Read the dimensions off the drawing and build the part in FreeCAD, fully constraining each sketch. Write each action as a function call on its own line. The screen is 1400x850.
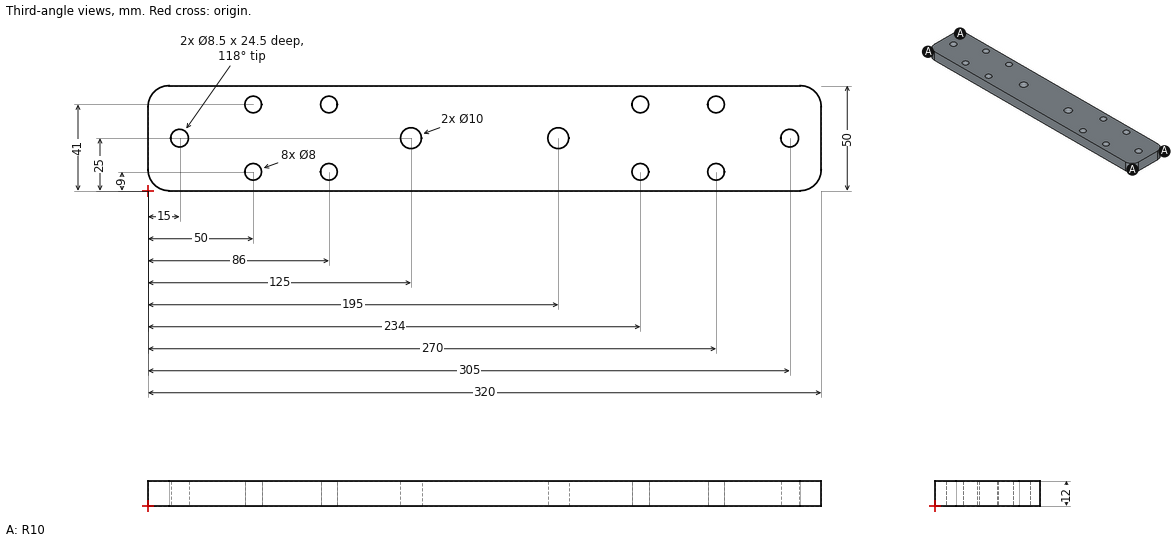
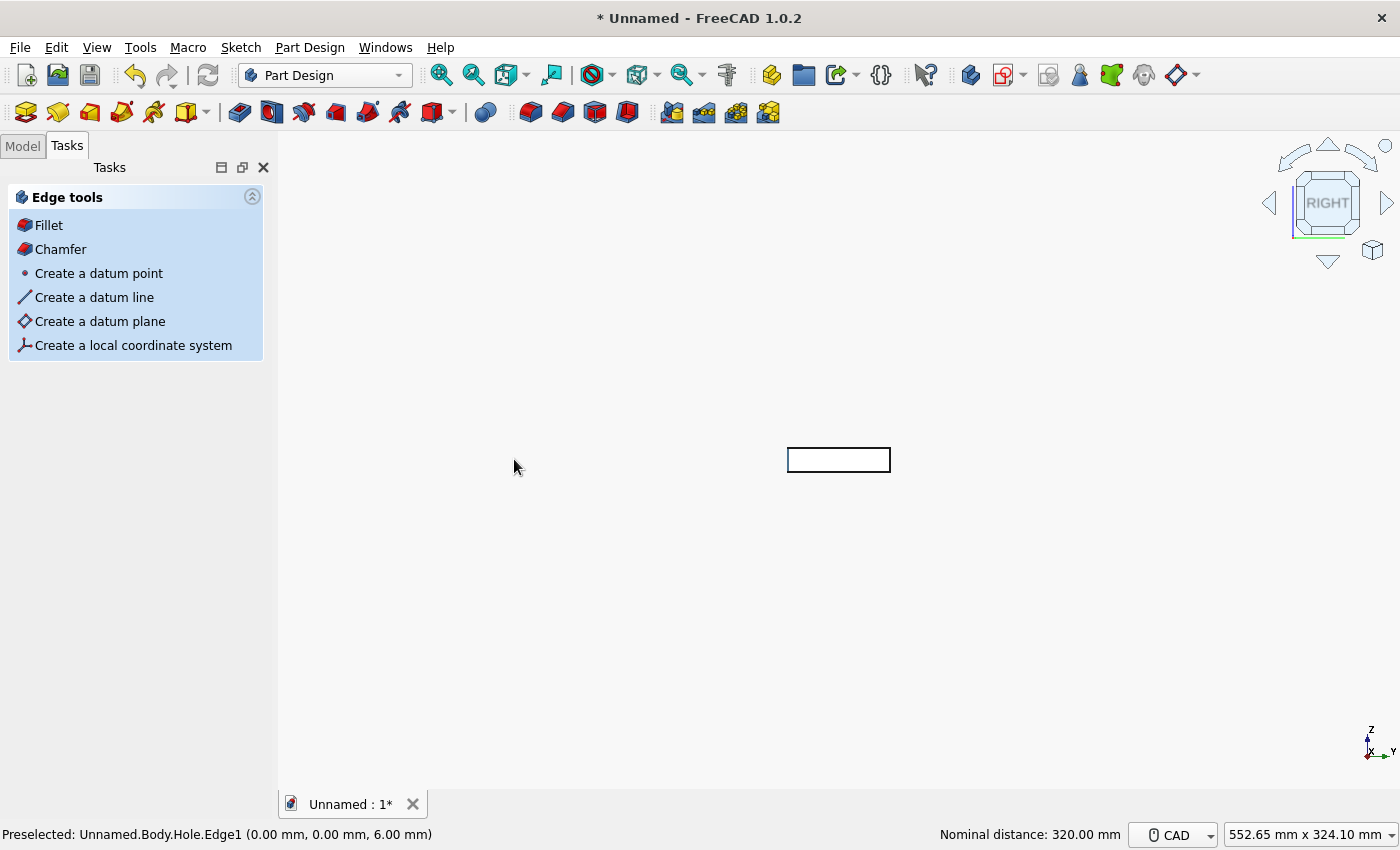
click(442, 76)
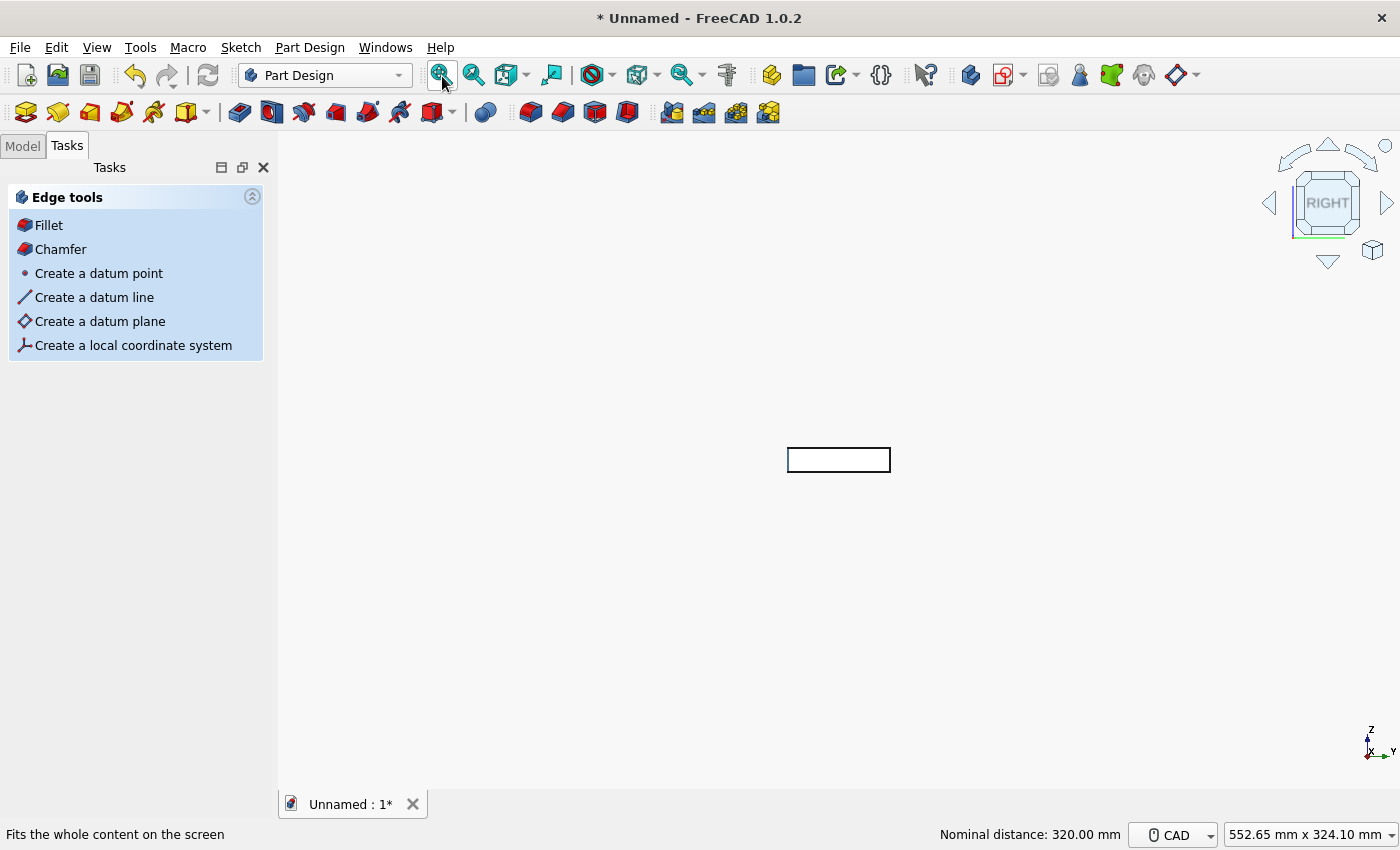
click(890, 459, ctrl)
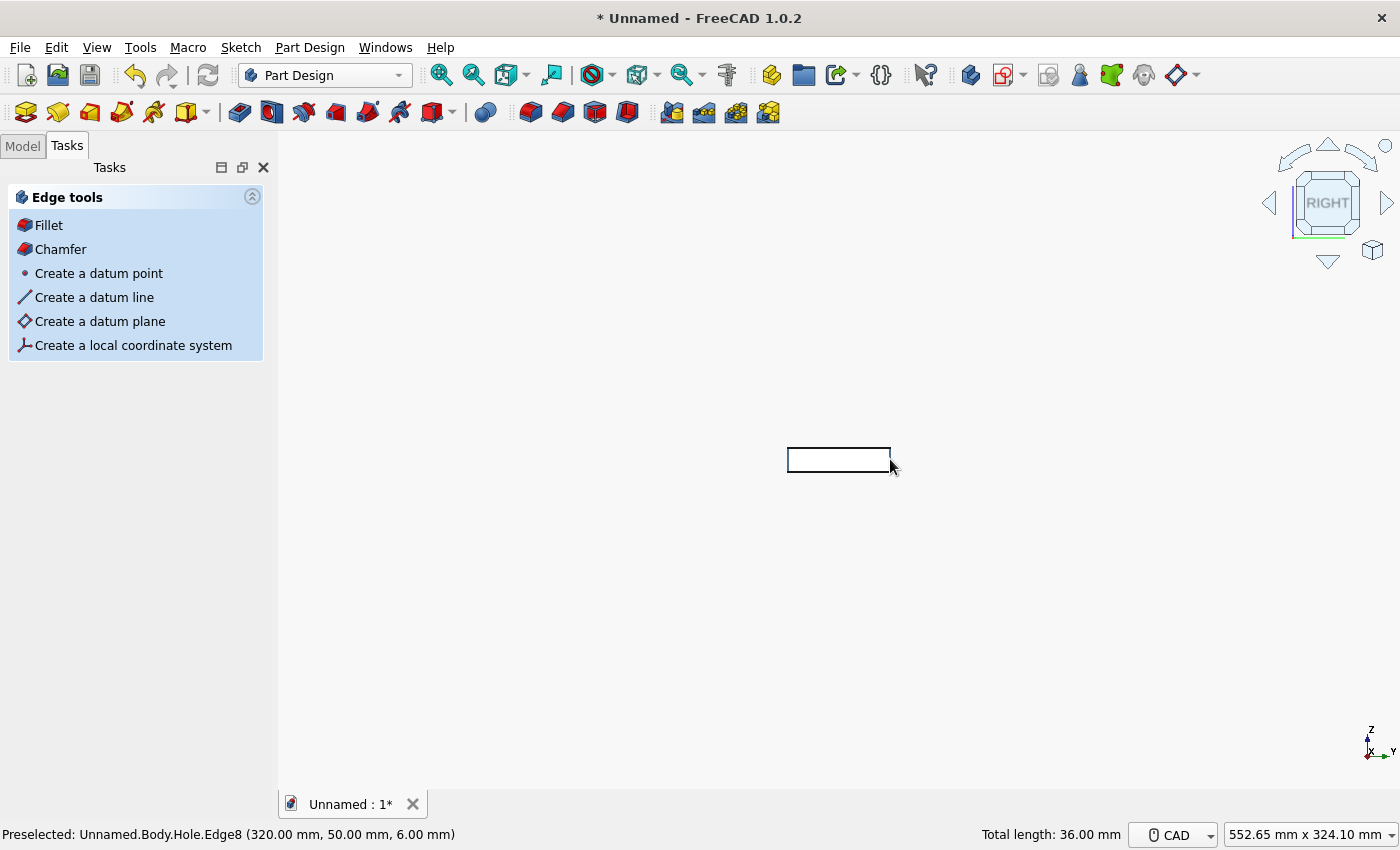
key(5)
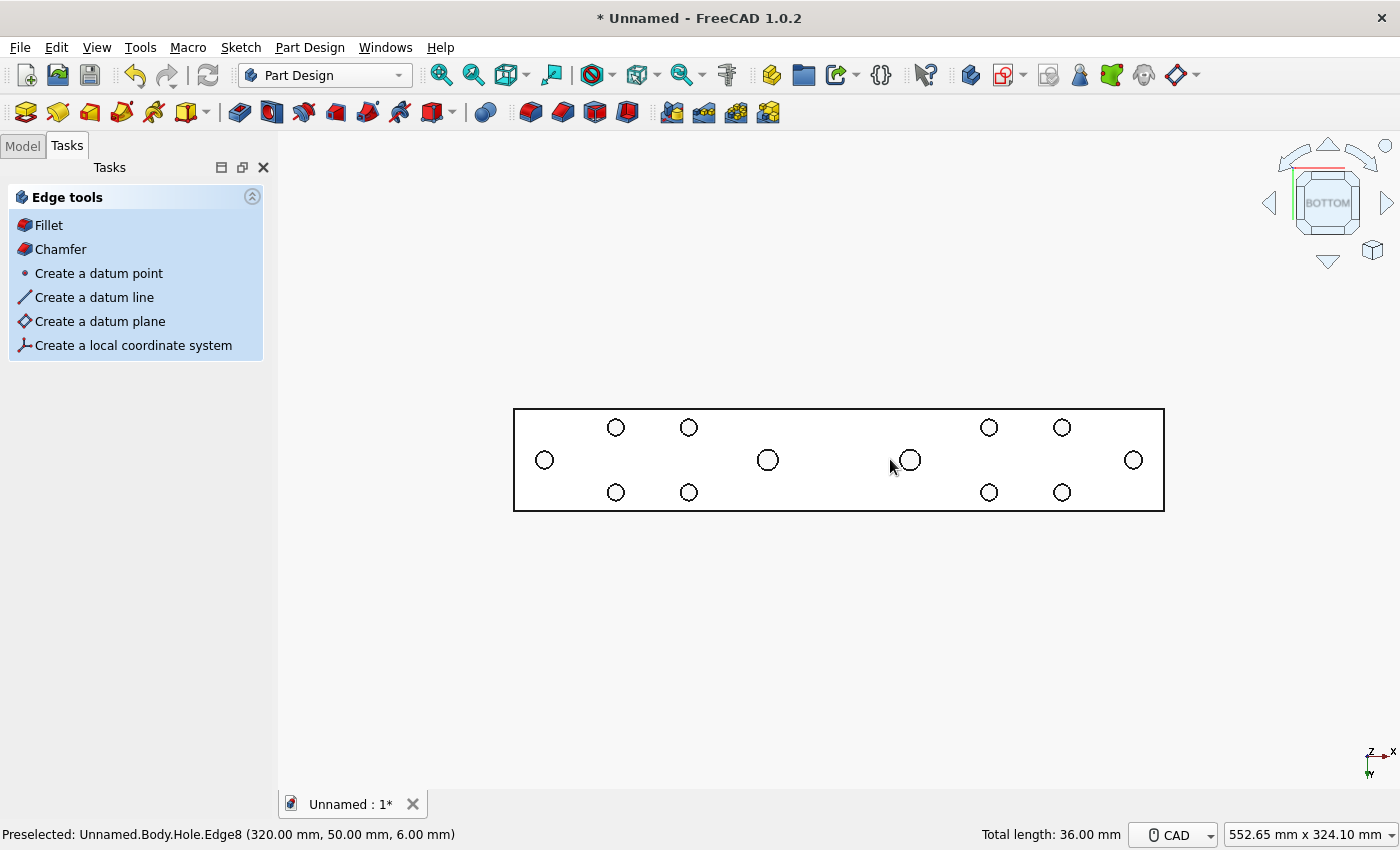
key(4)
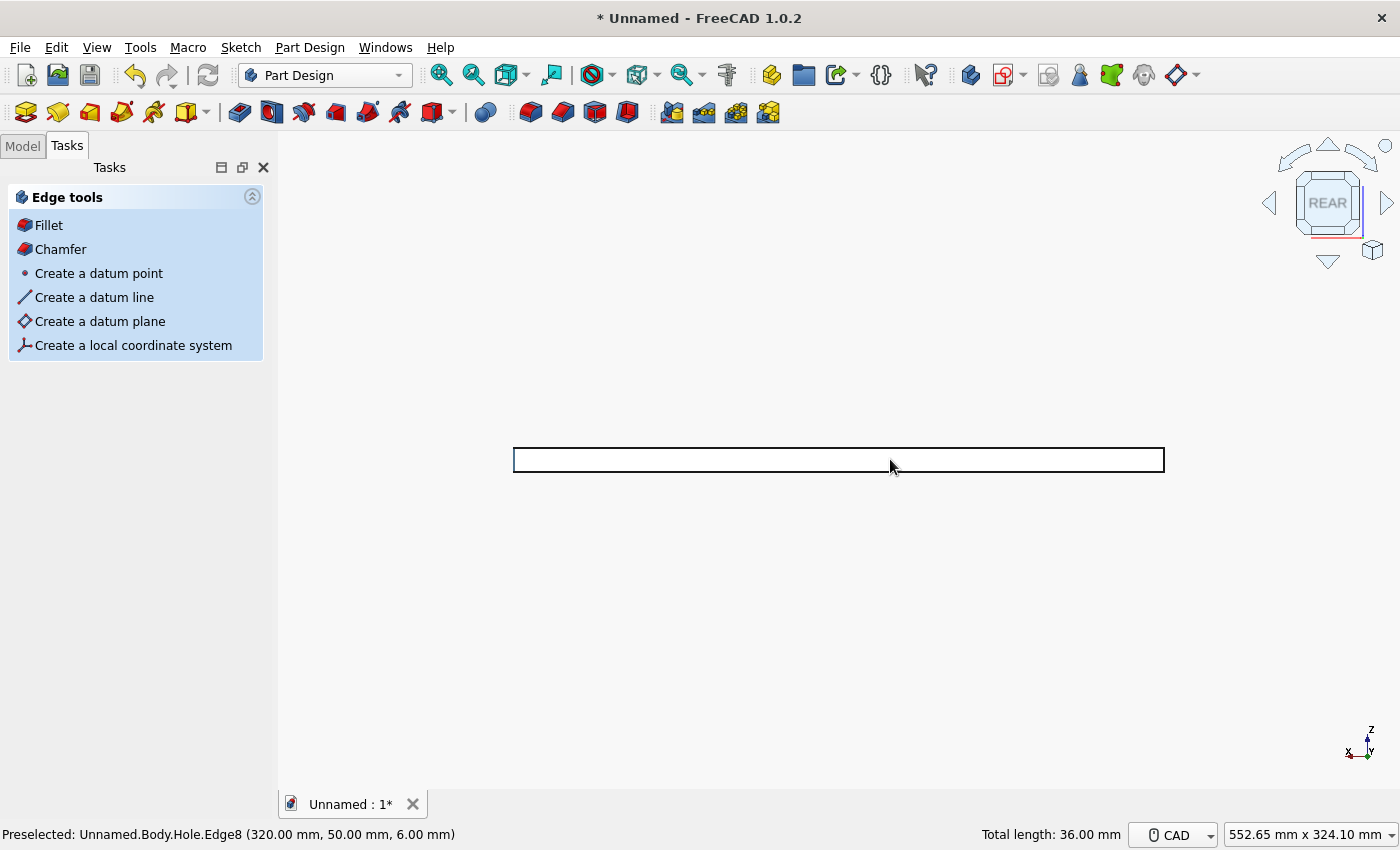
click(1164, 459, ctrl)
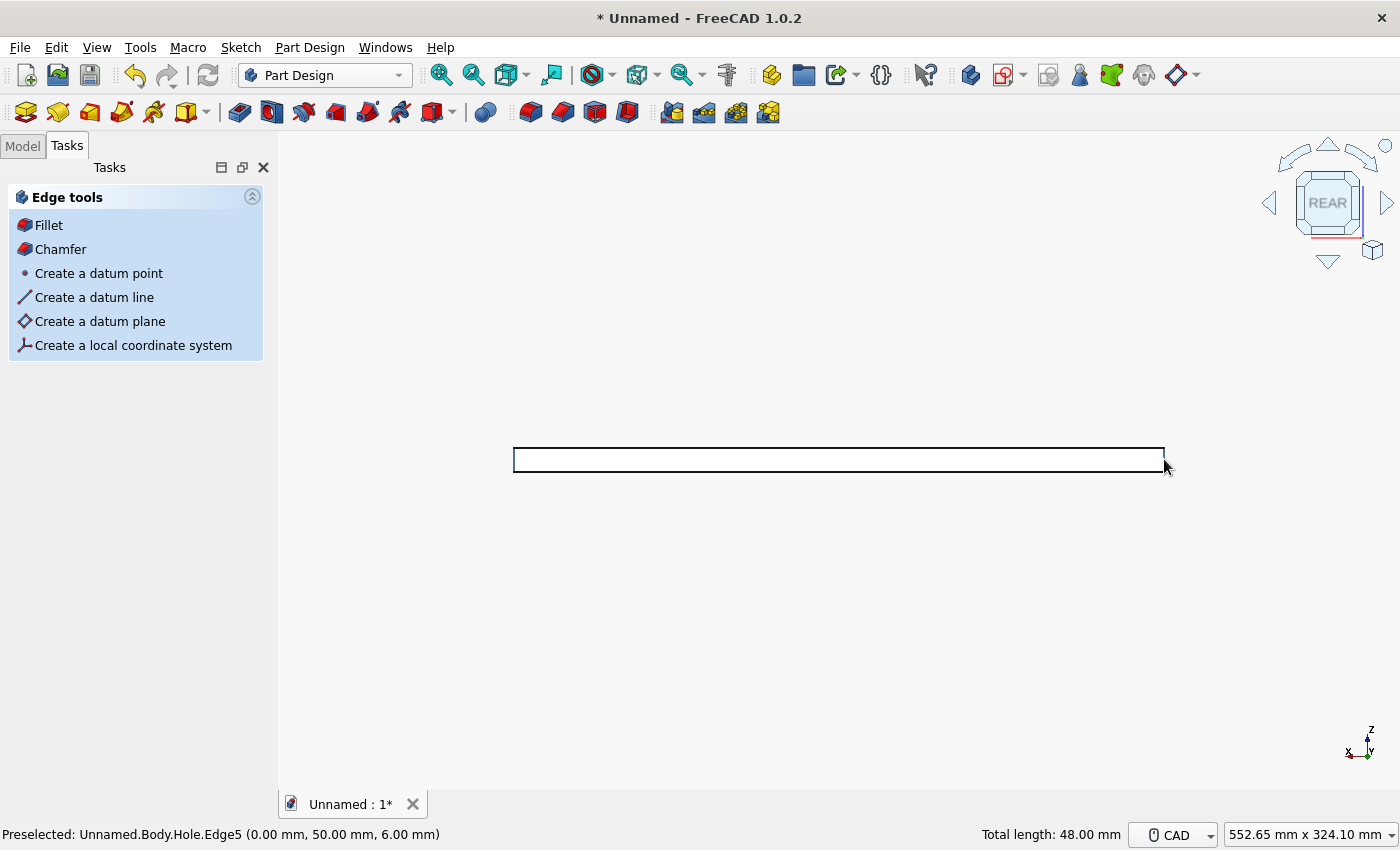
click(532, 112)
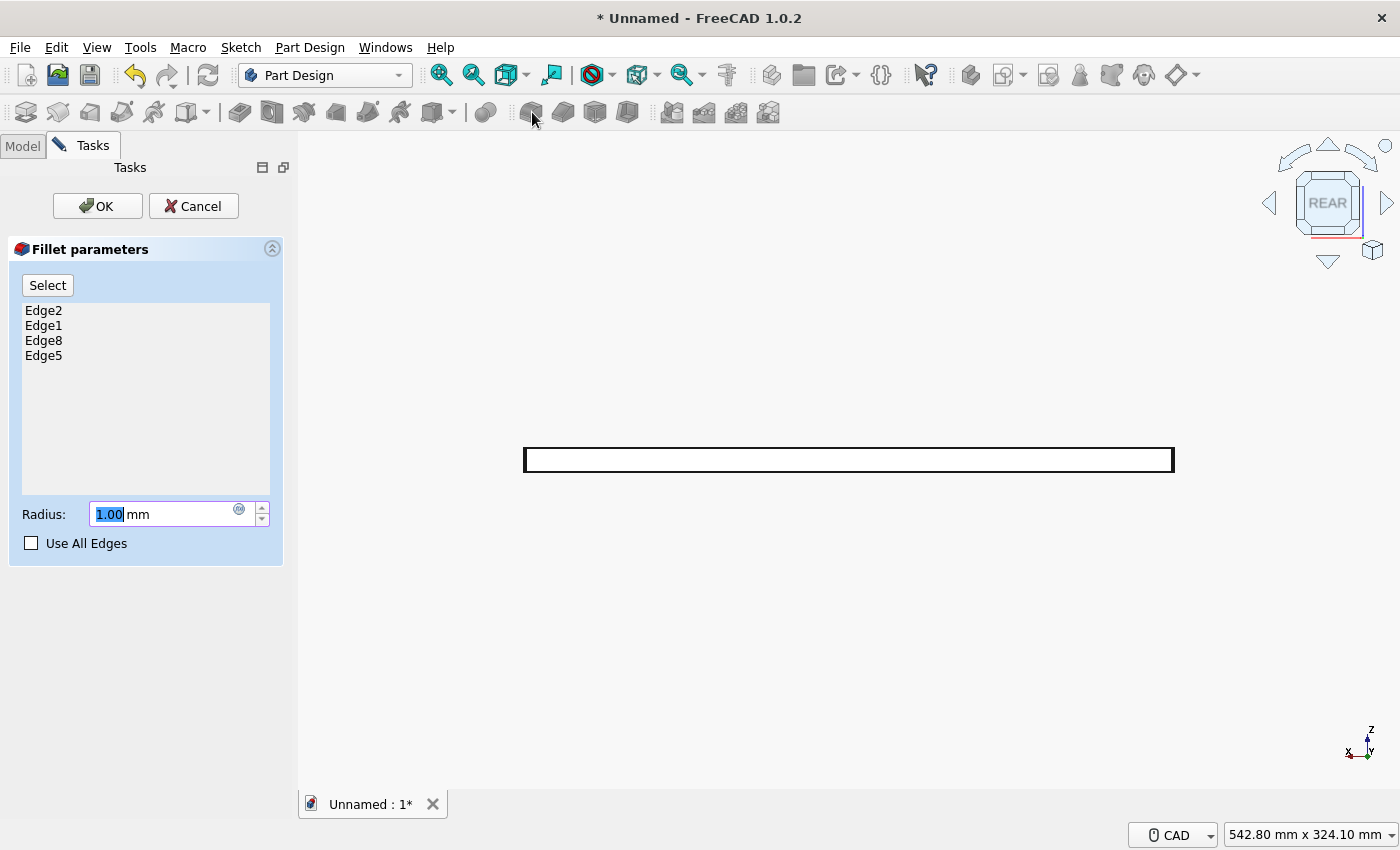
text(10)
key(Tab)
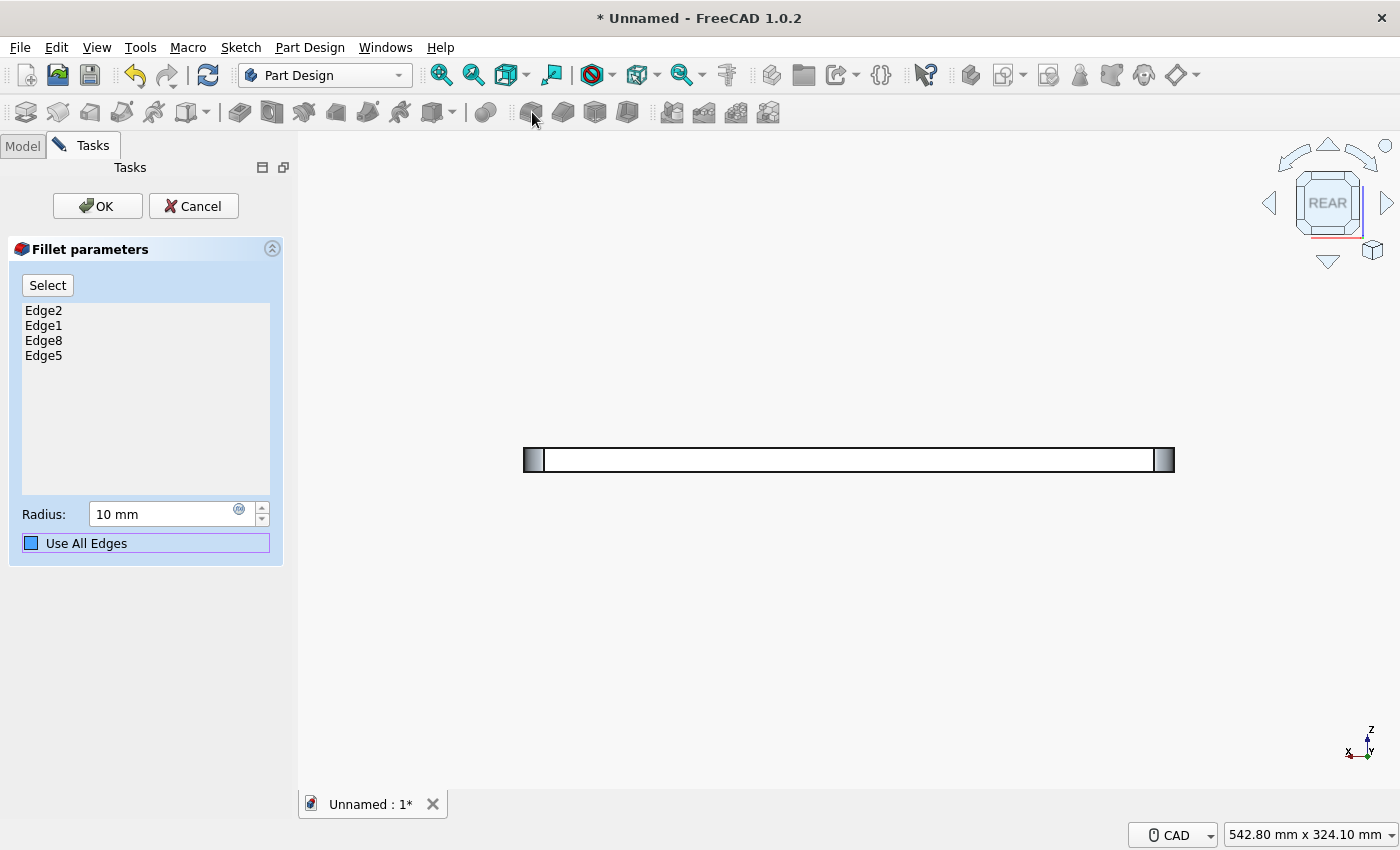
click(98, 206)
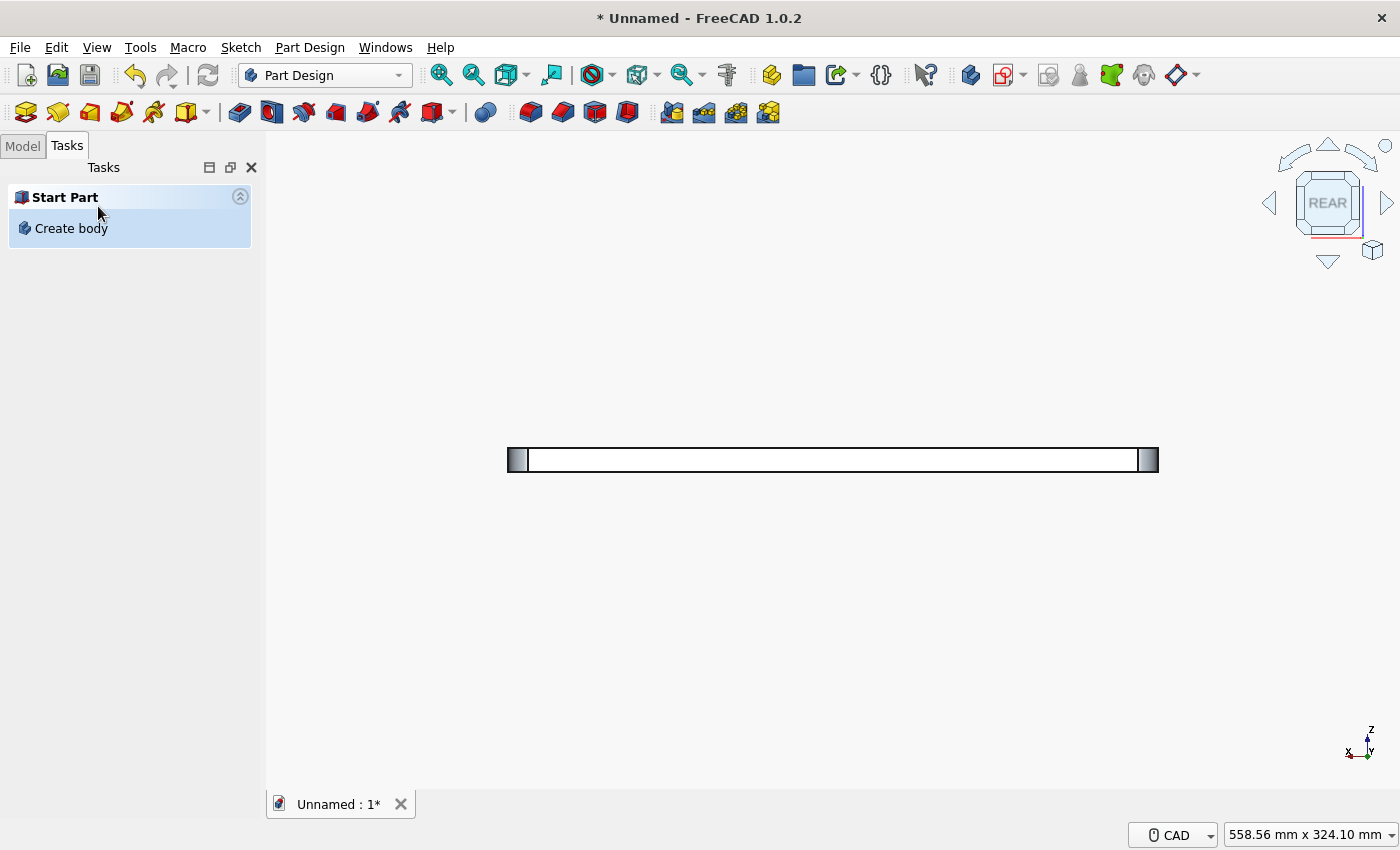
key(0)